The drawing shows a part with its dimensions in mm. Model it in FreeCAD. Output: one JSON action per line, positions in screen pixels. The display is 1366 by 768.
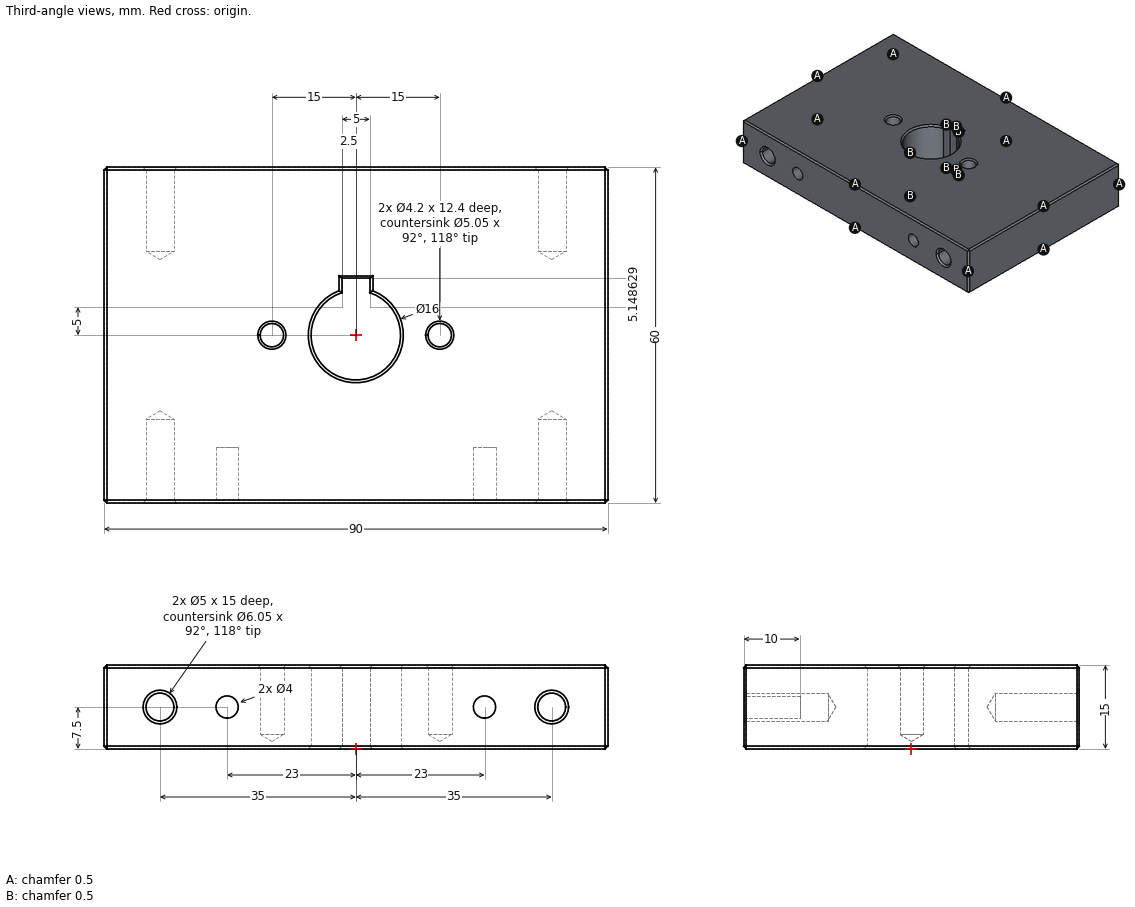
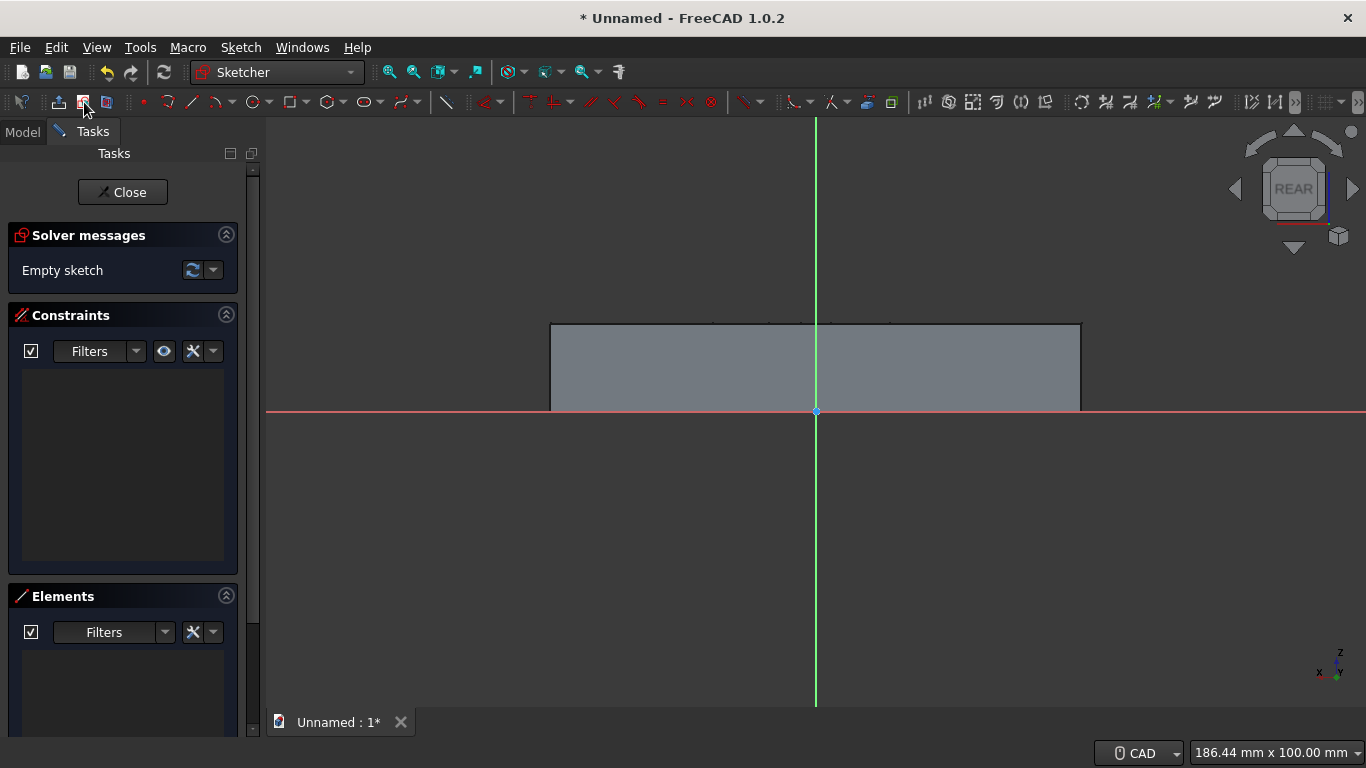
{"action": "scroll", "coordinate": [955, 323], "scroll_direction": "up", "scroll_amount": 2}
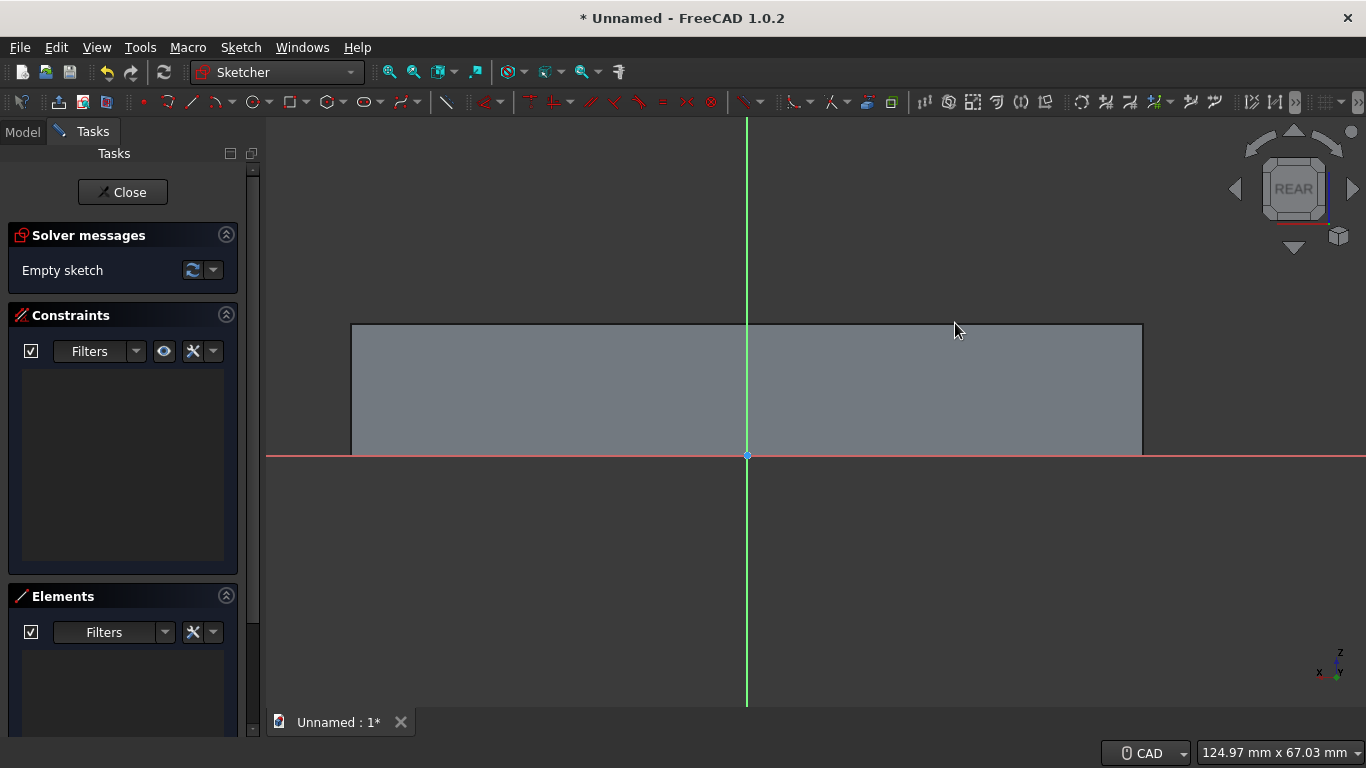
{"action": "key", "text": "g c"}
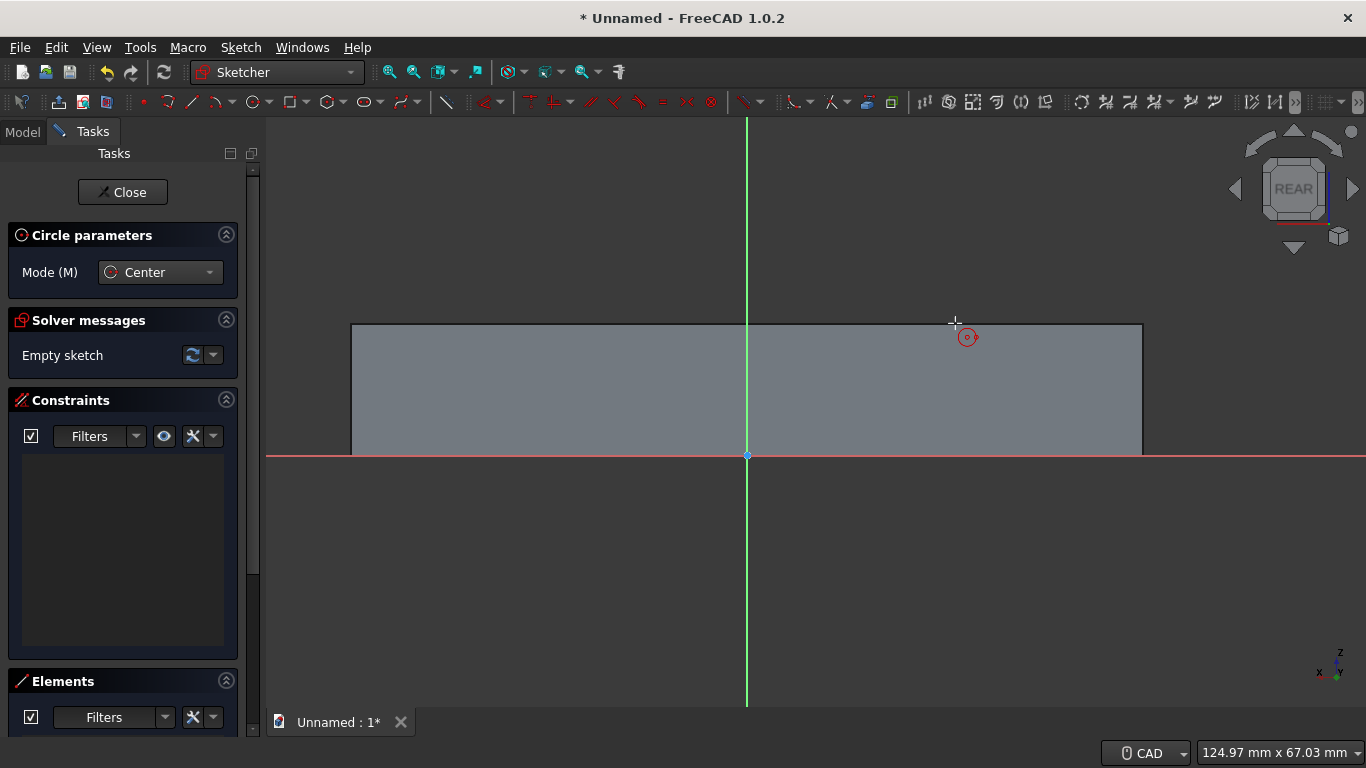
{"action": "left_click", "coordinate": [1055, 390]}
{"action": "mouse_move", "coordinate": [1071, 374]}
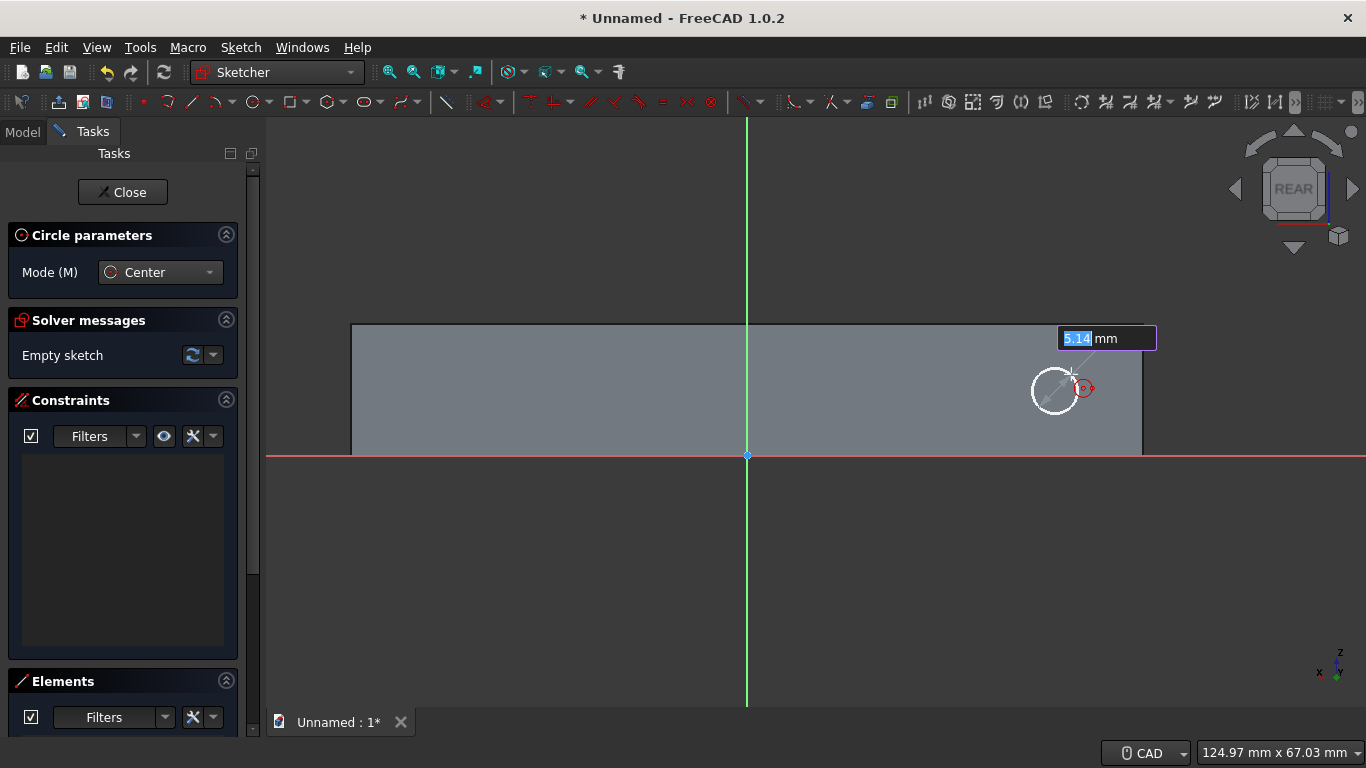
{"action": "type", "text": "5"}
{"action": "key", "text": "Return"}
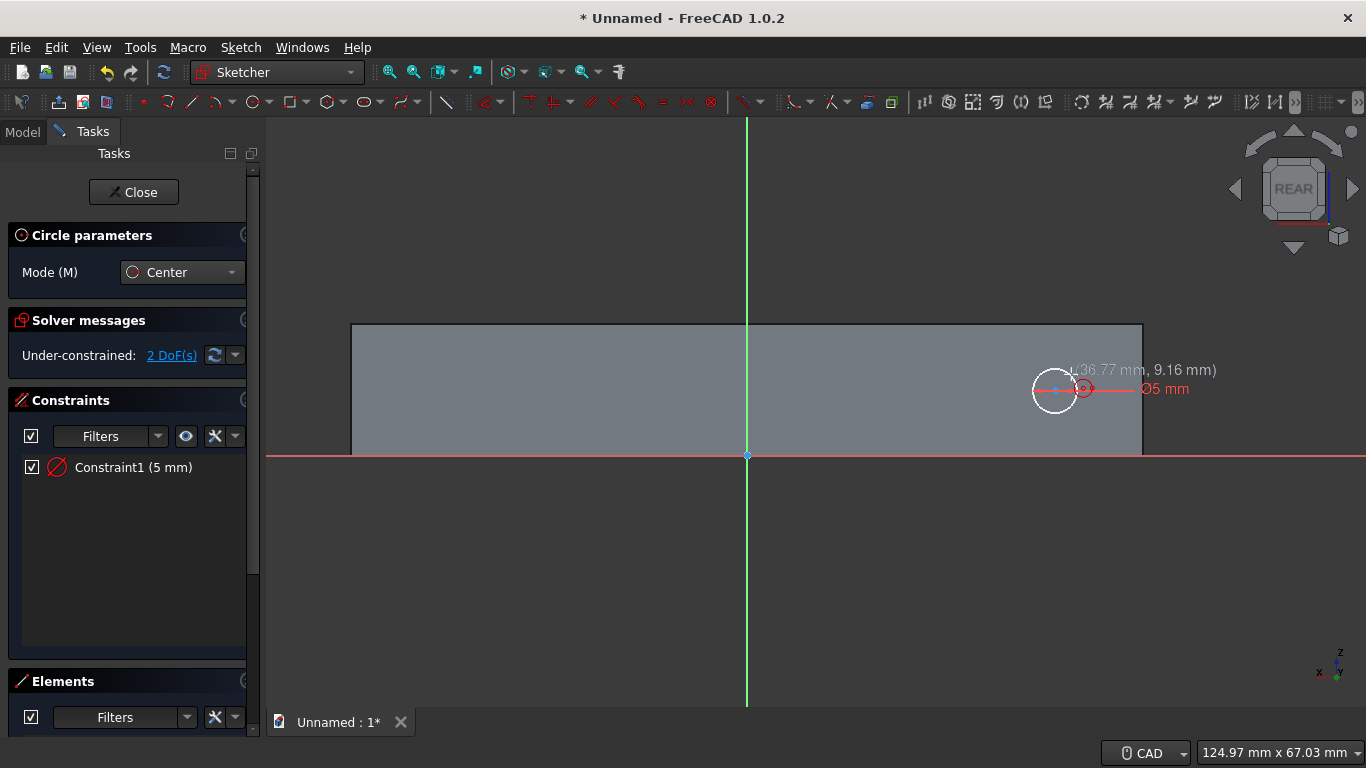
{"action": "left_click", "coordinate": [439, 390]}
{"action": "mouse_move", "coordinate": [455, 374]}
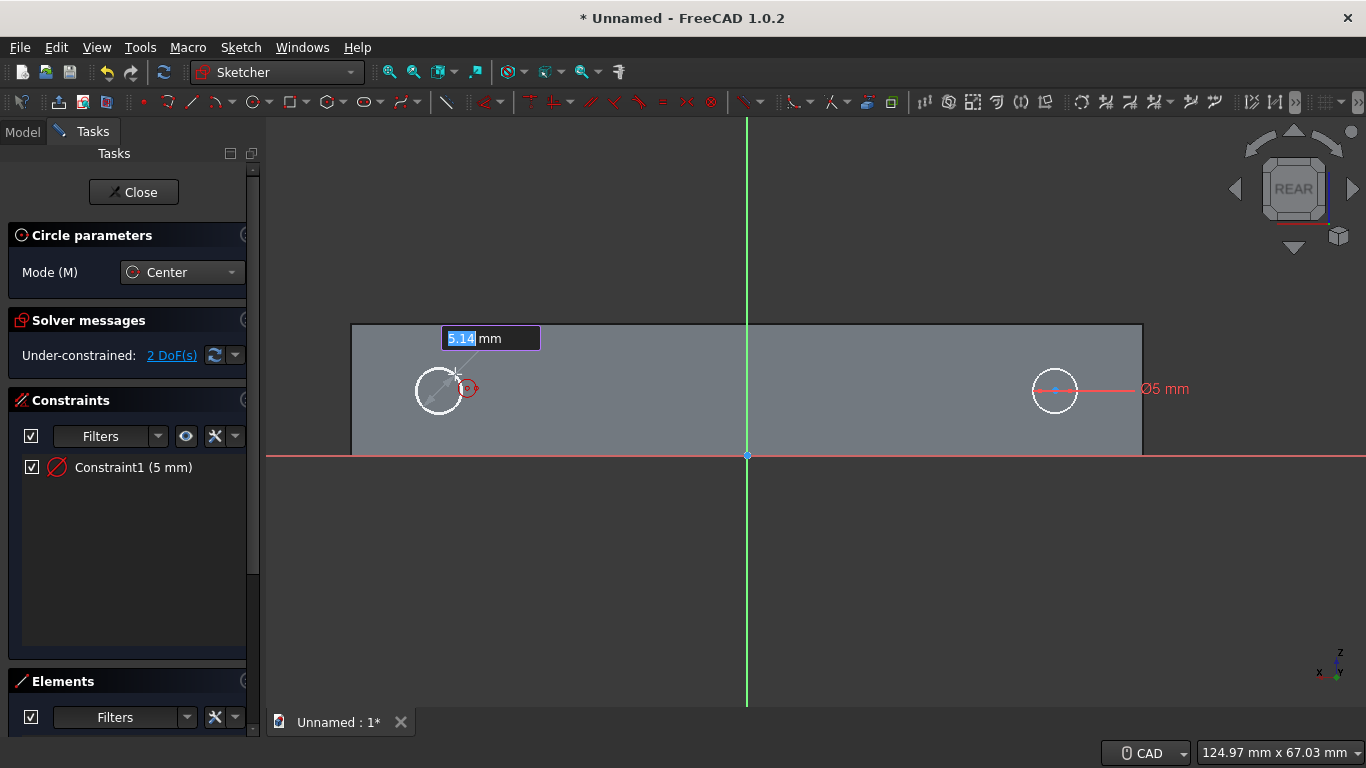
{"action": "type", "text": "5"}
{"action": "key", "text": "Return"}
{"action": "key", "text": "Escape"}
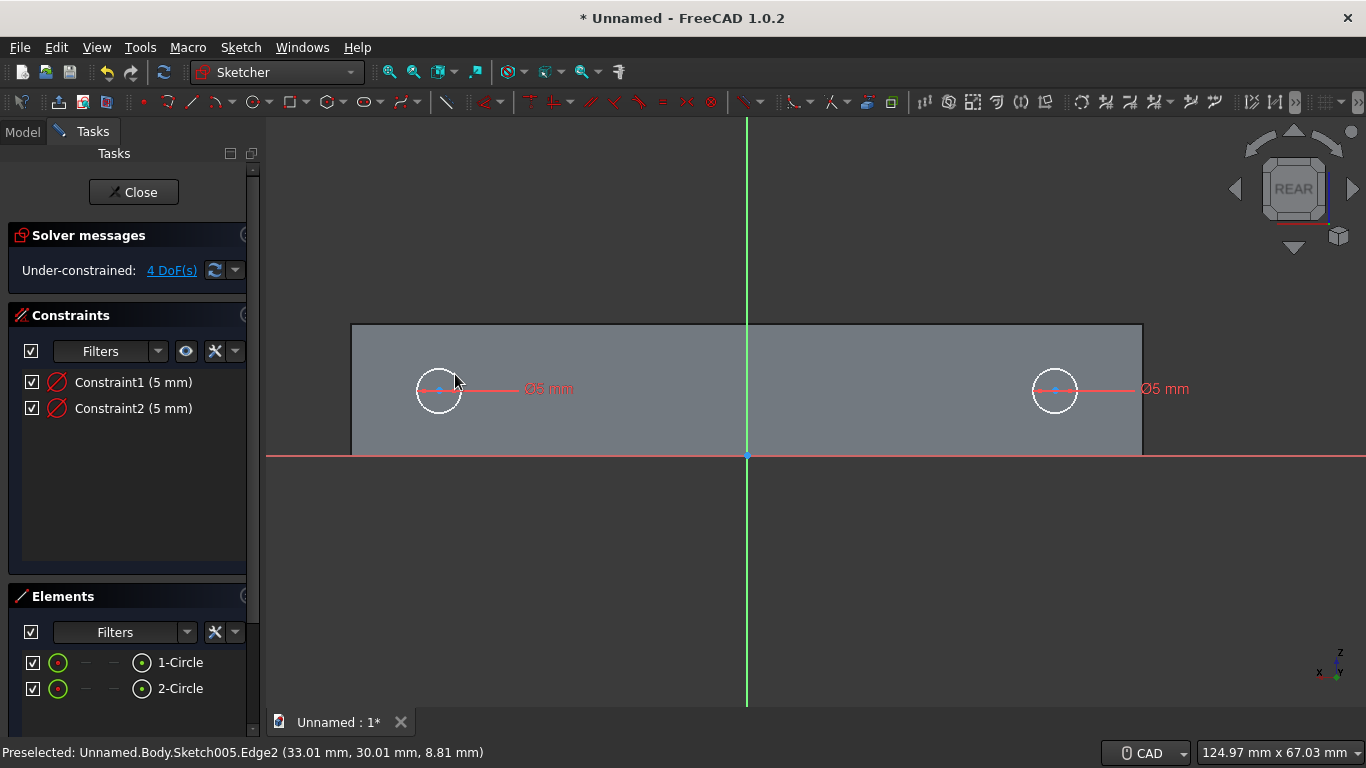
{"action": "left_click", "coordinate": [1055, 391]}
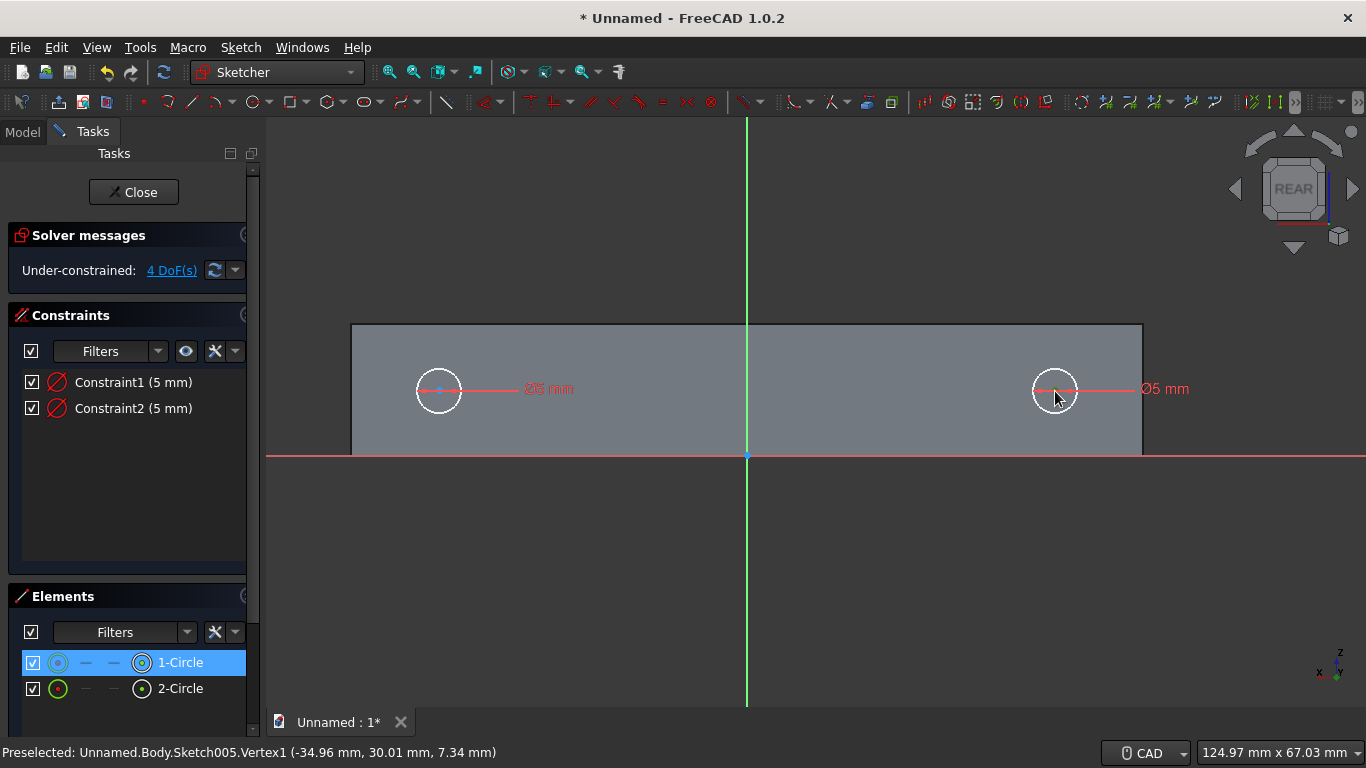
{"action": "left_click", "coordinate": [439, 391]}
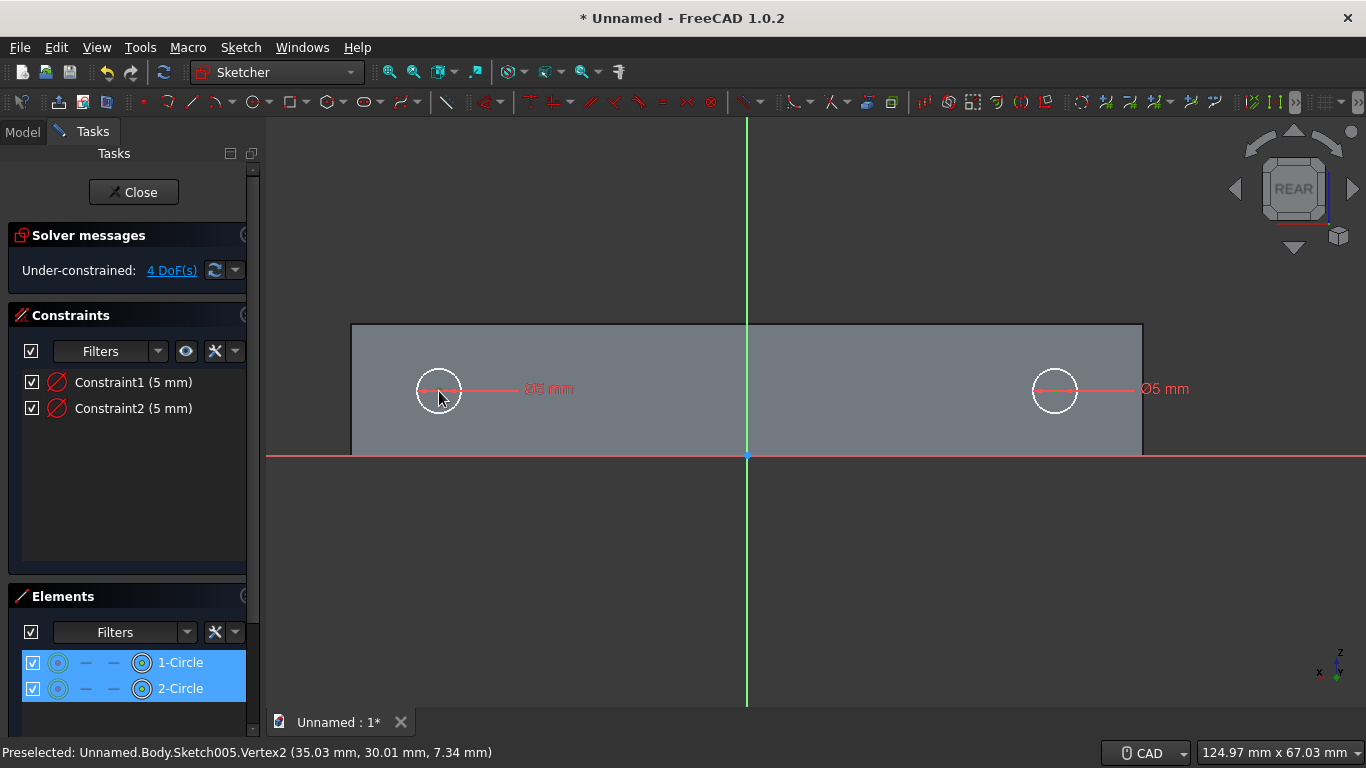
{"action": "key", "text": "h"}